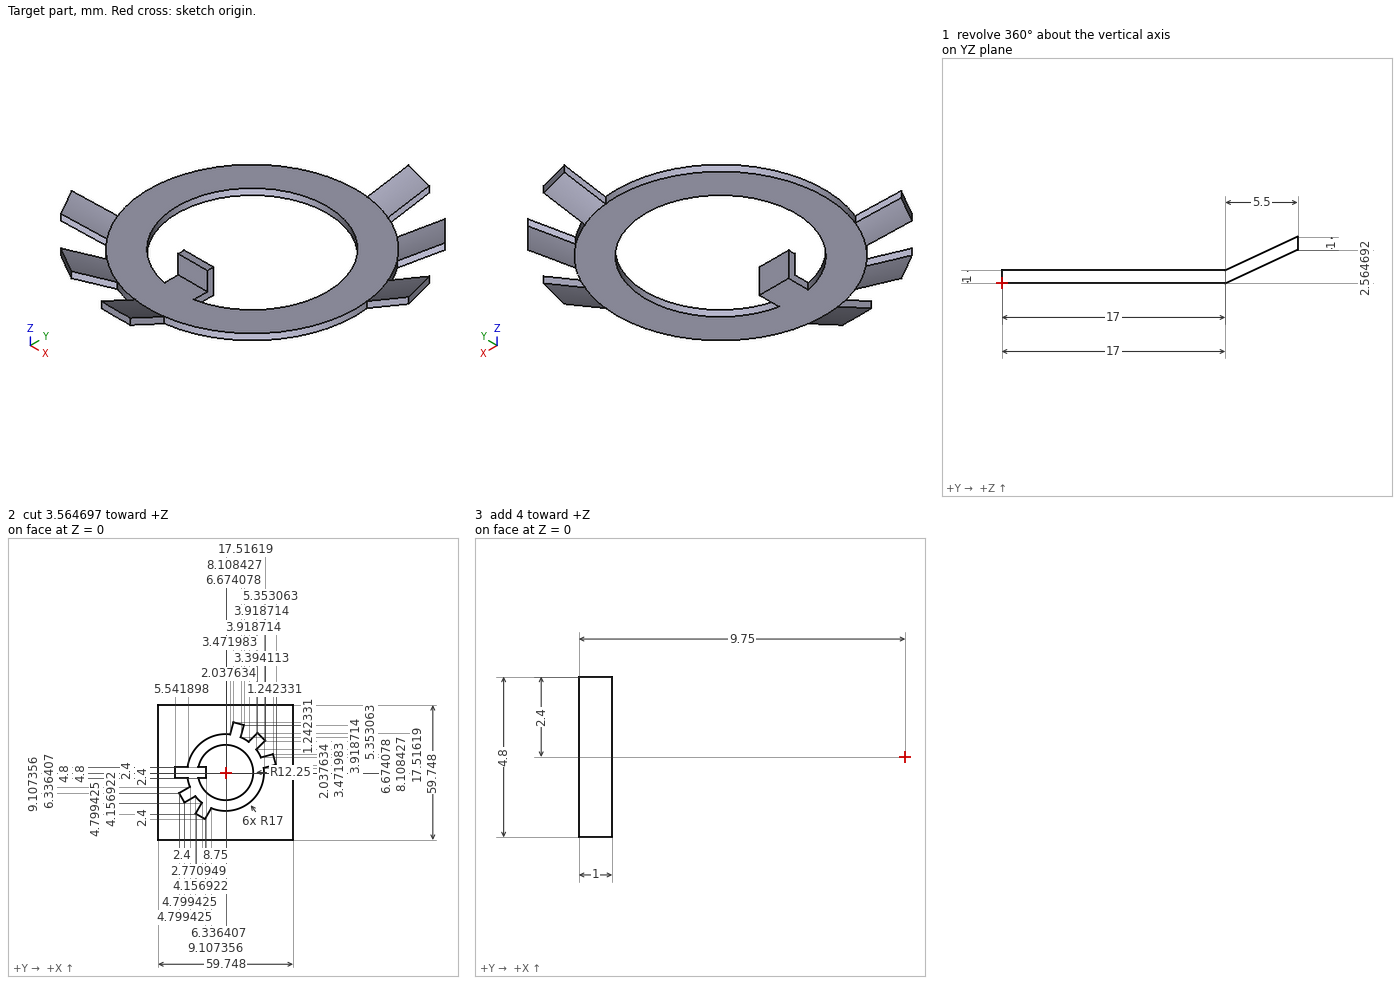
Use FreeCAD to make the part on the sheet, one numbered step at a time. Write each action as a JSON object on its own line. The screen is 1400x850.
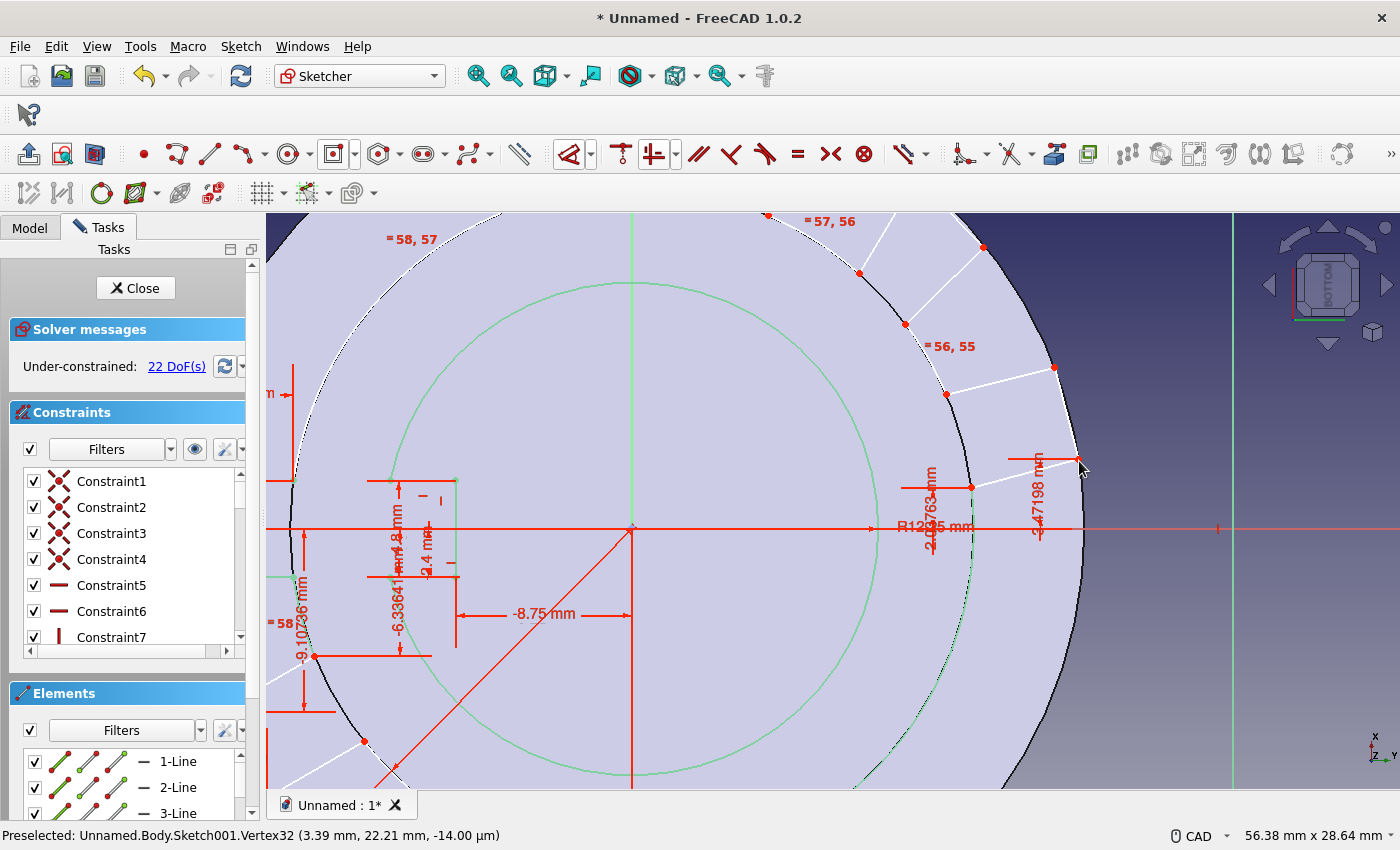
{"action": "left_click", "coordinate": [1055, 368]}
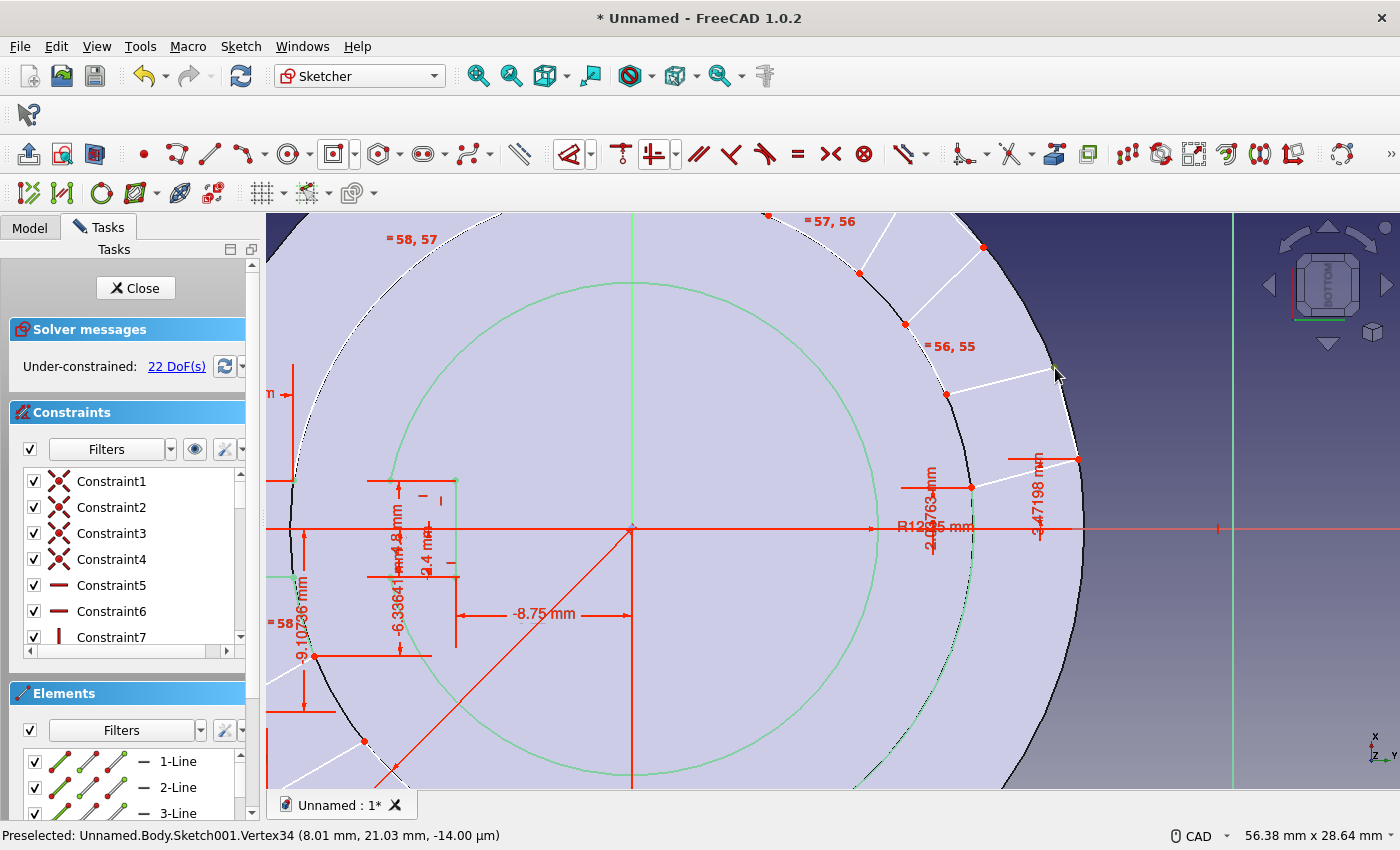
{"action": "left_click", "coordinate": [590, 154]}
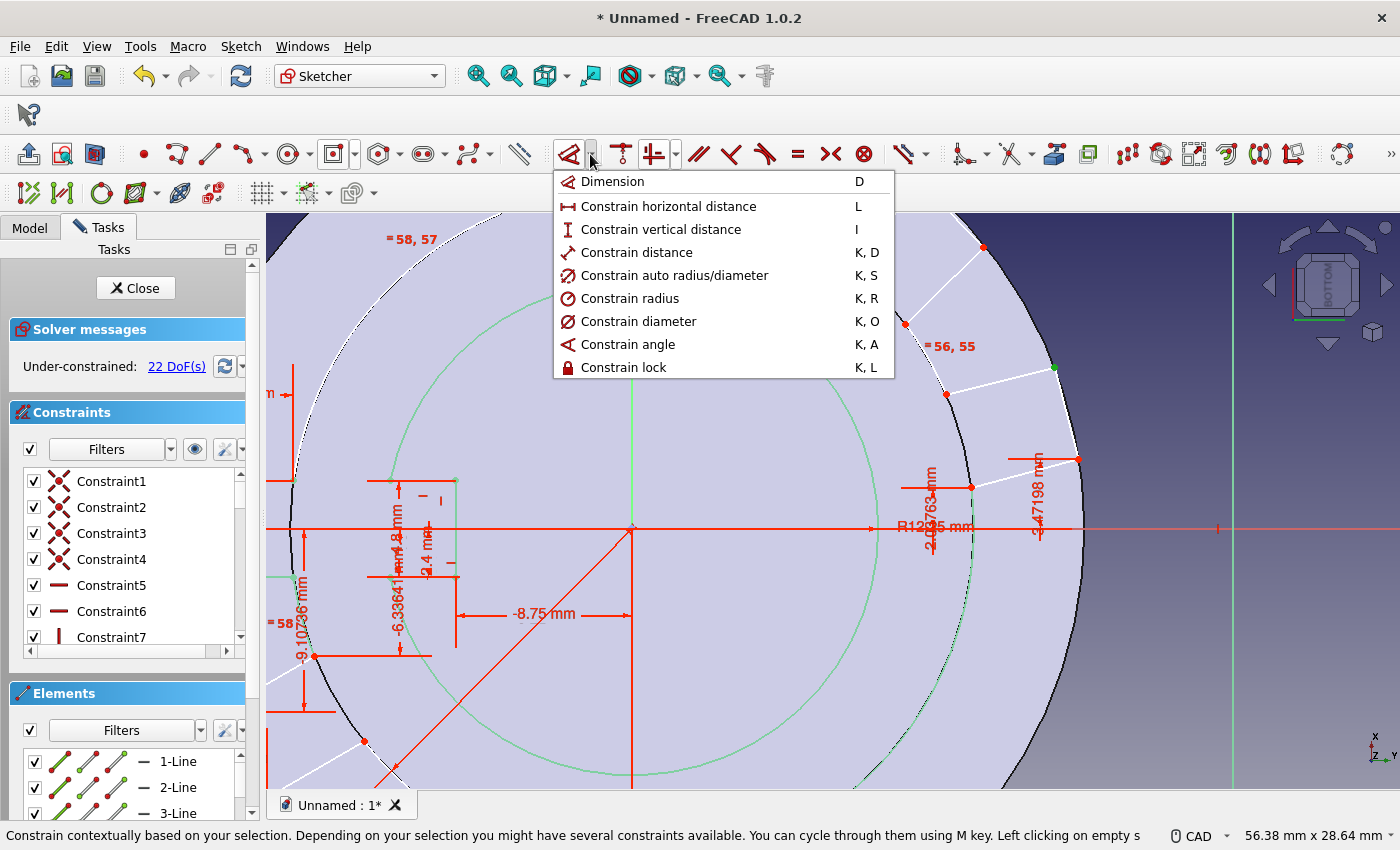
{"action": "left_click", "coordinate": [724, 230]}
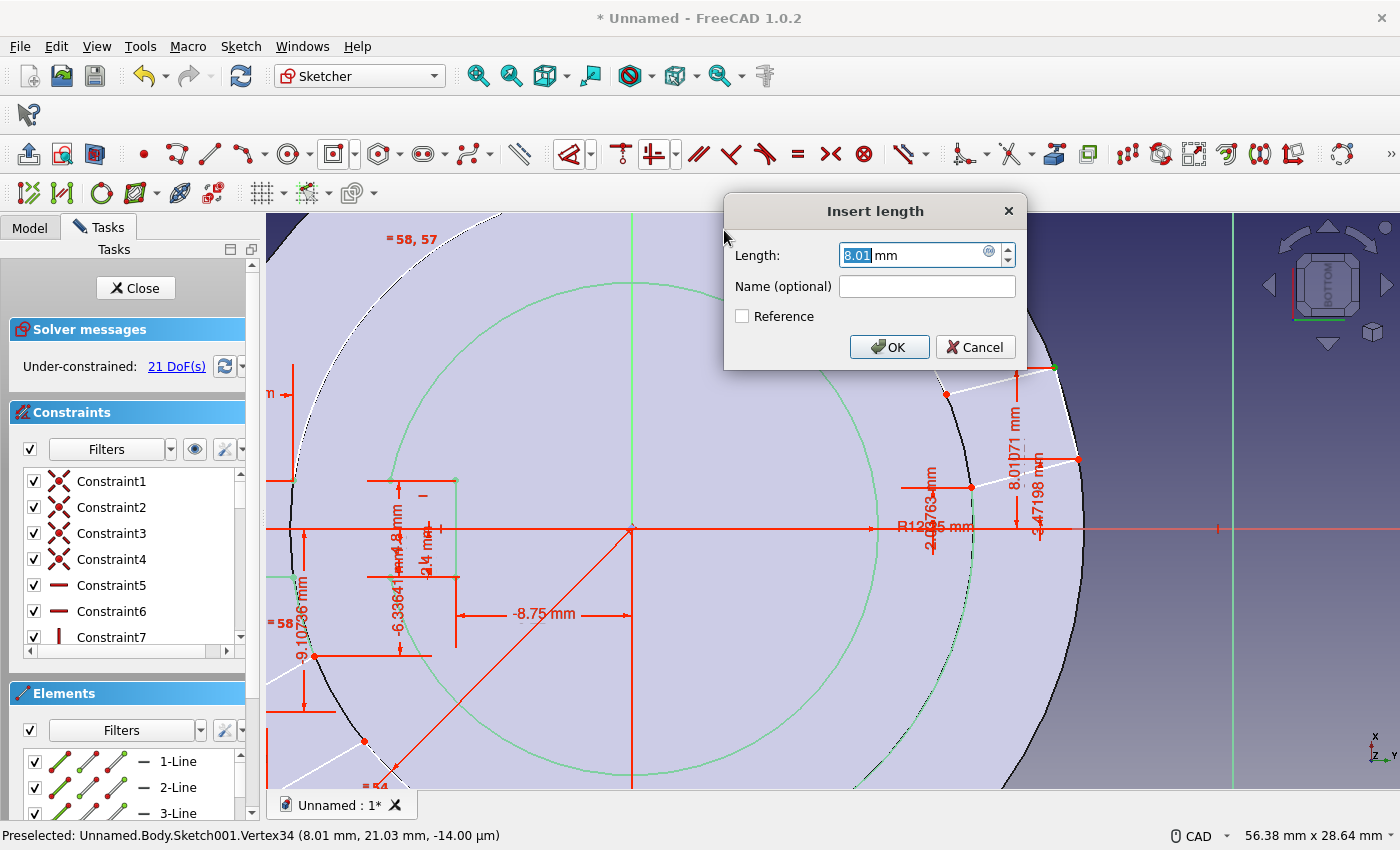
{"action": "type", "text": "8.108427"}
{"action": "key", "text": "Return"}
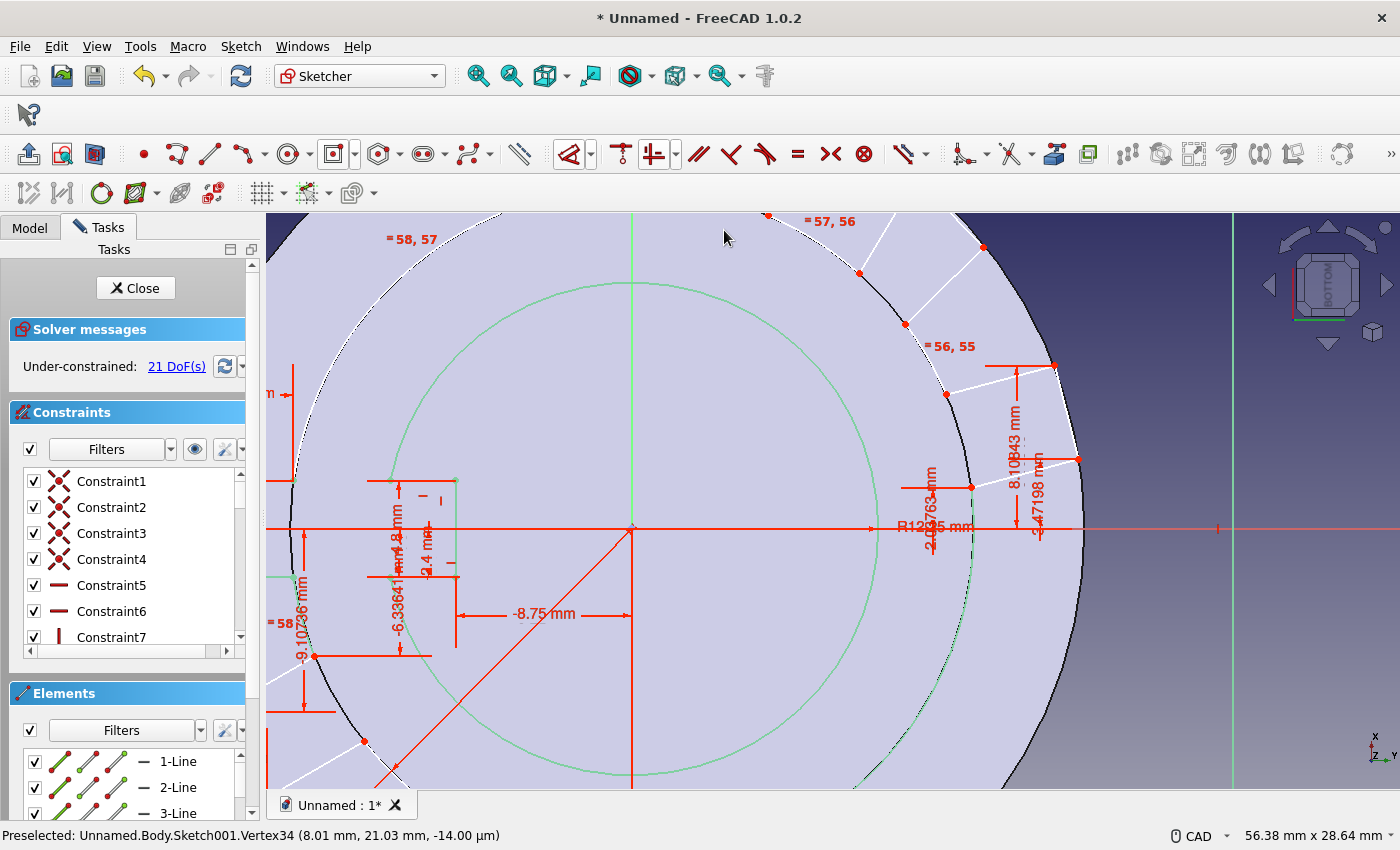
{"action": "left_click", "coordinate": [946, 395]}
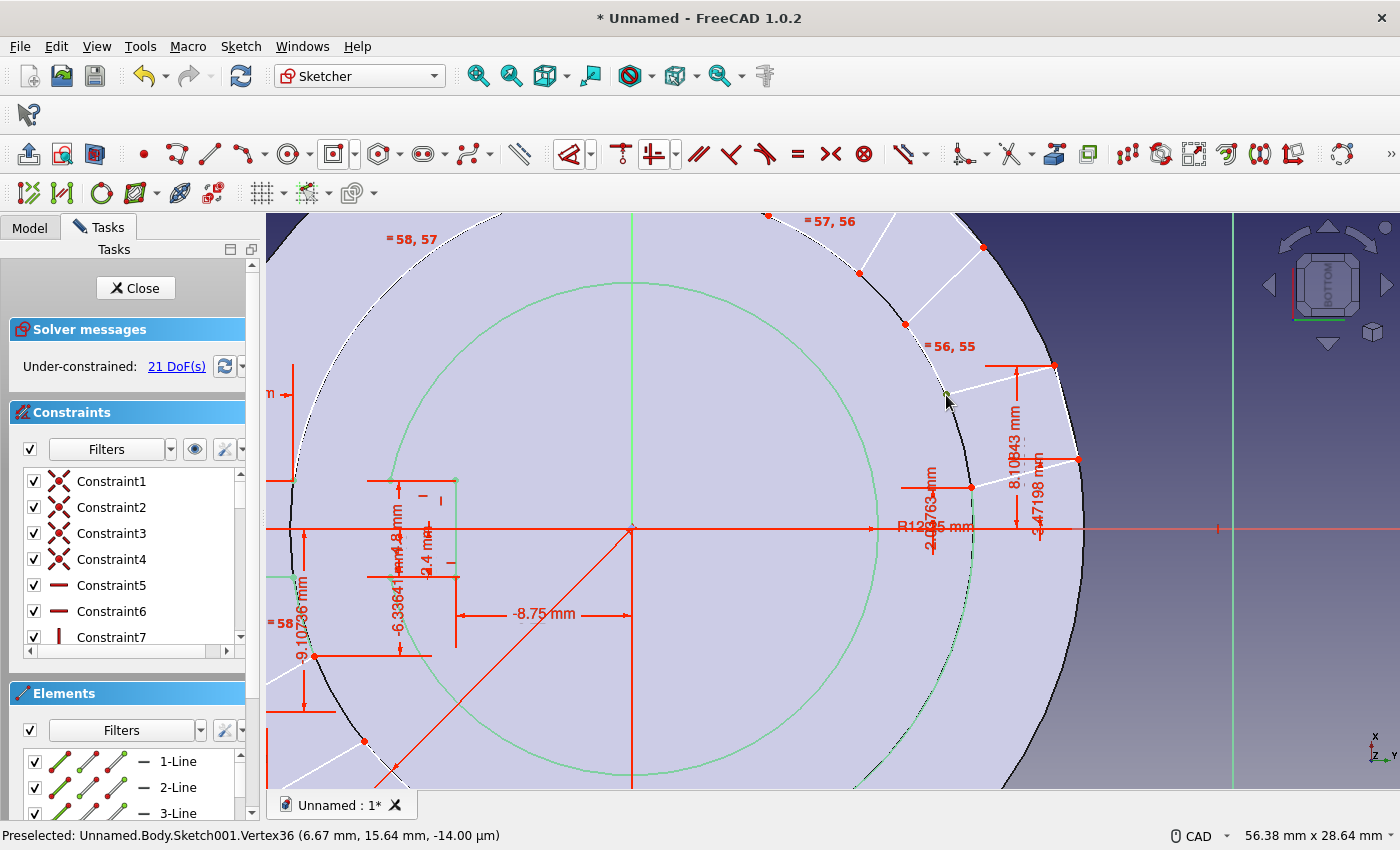
{"action": "key", "text": "i"}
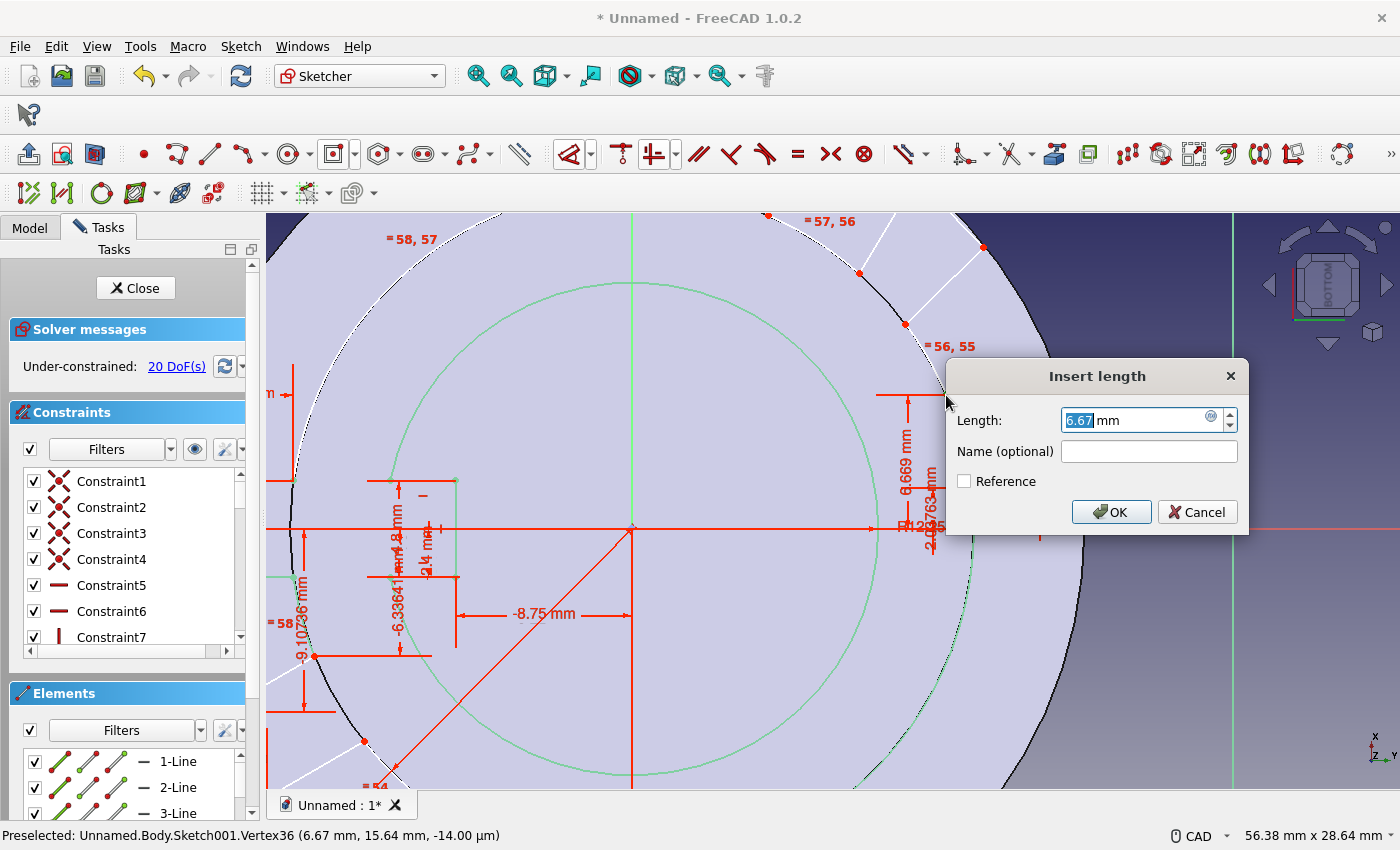
{"action": "type", "text": "6.674078"}
{"action": "key", "text": "Return"}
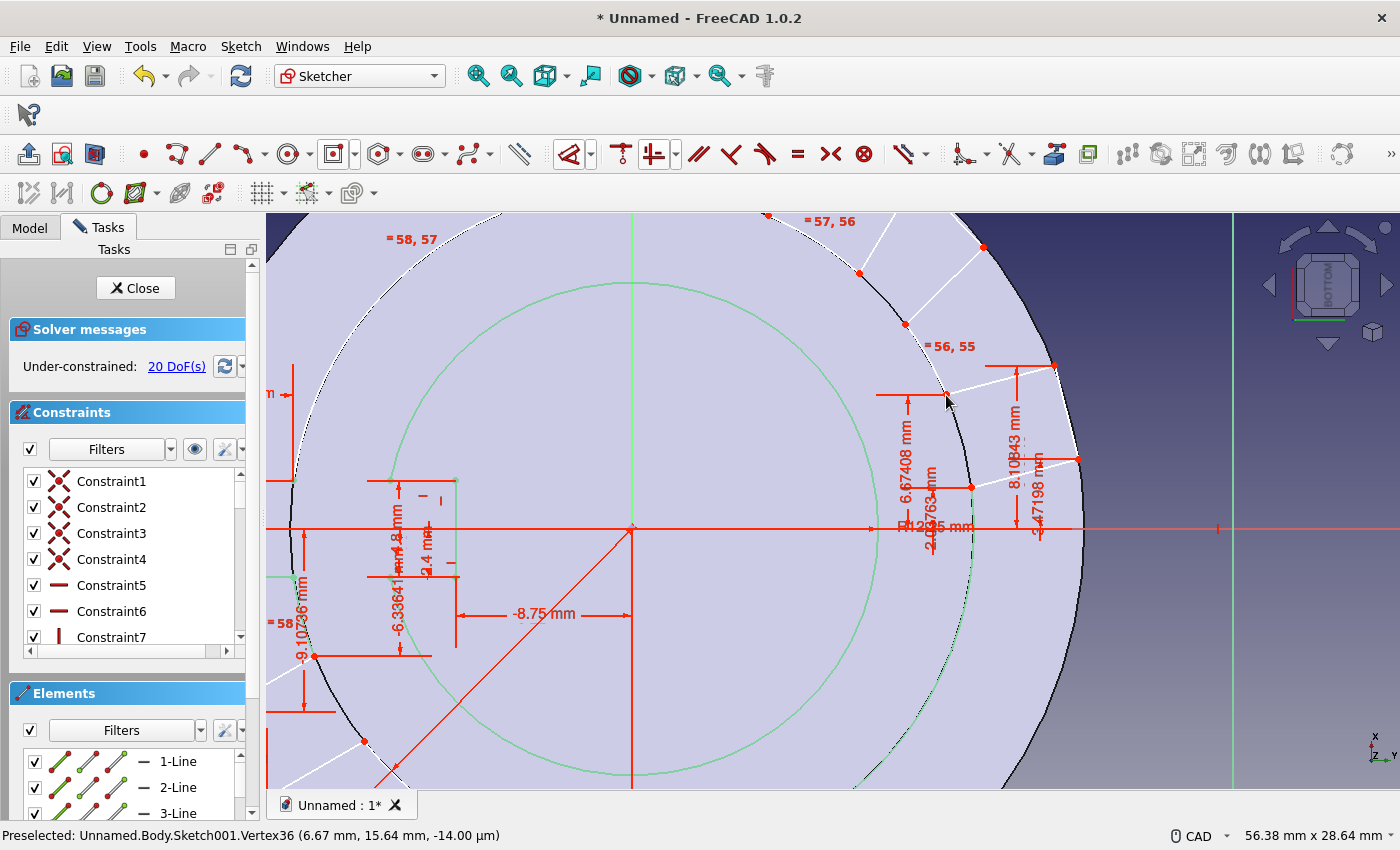
{"action": "left_click", "coordinate": [984, 248]}